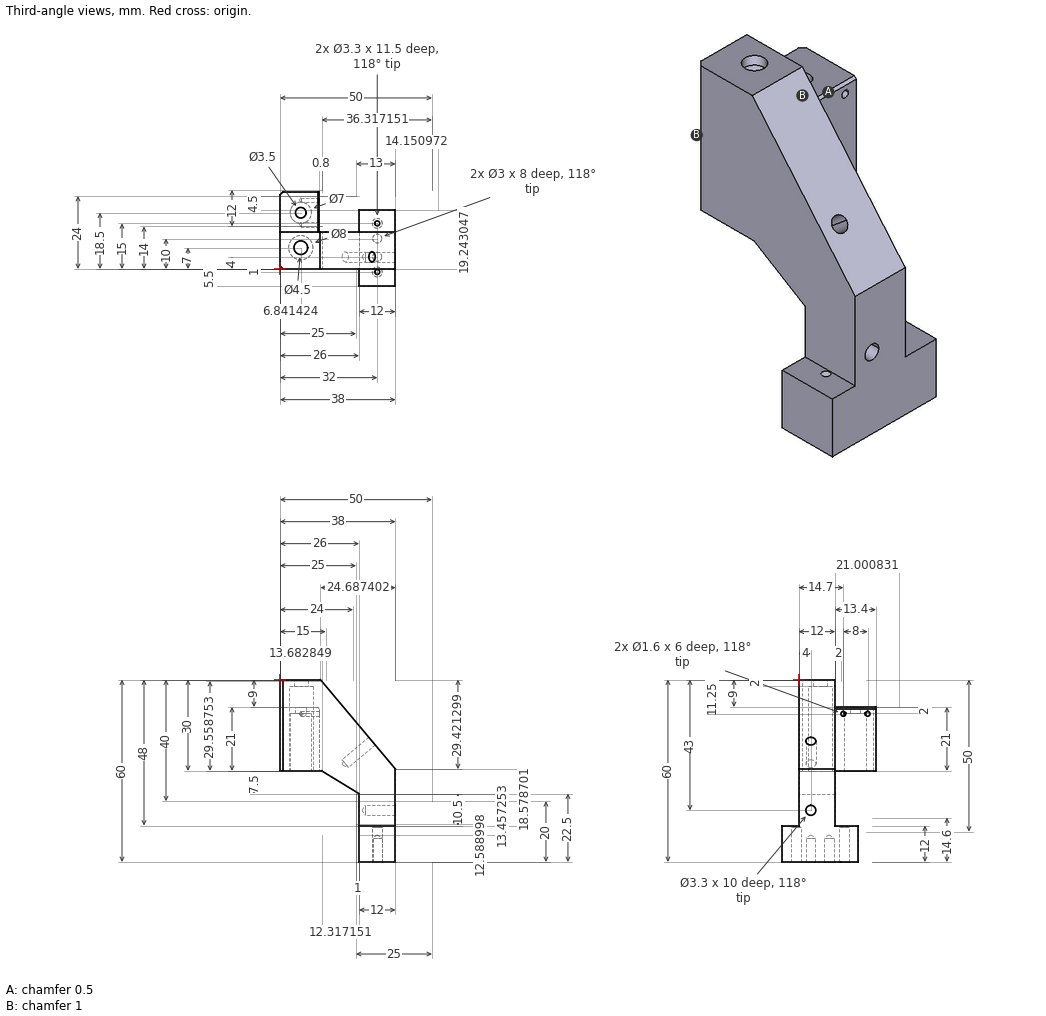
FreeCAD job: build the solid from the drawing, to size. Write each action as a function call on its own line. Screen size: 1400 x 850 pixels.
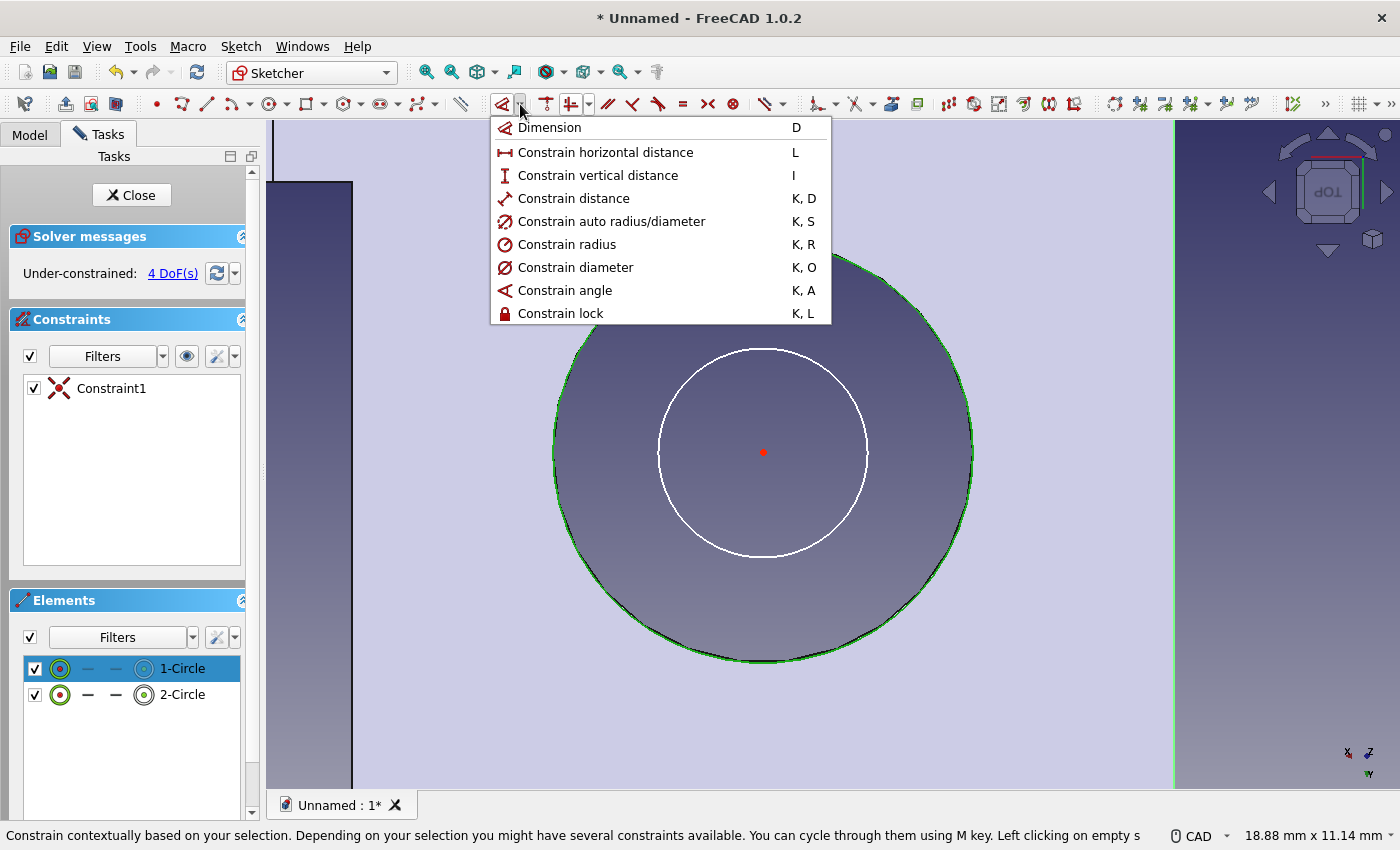
click(661, 268)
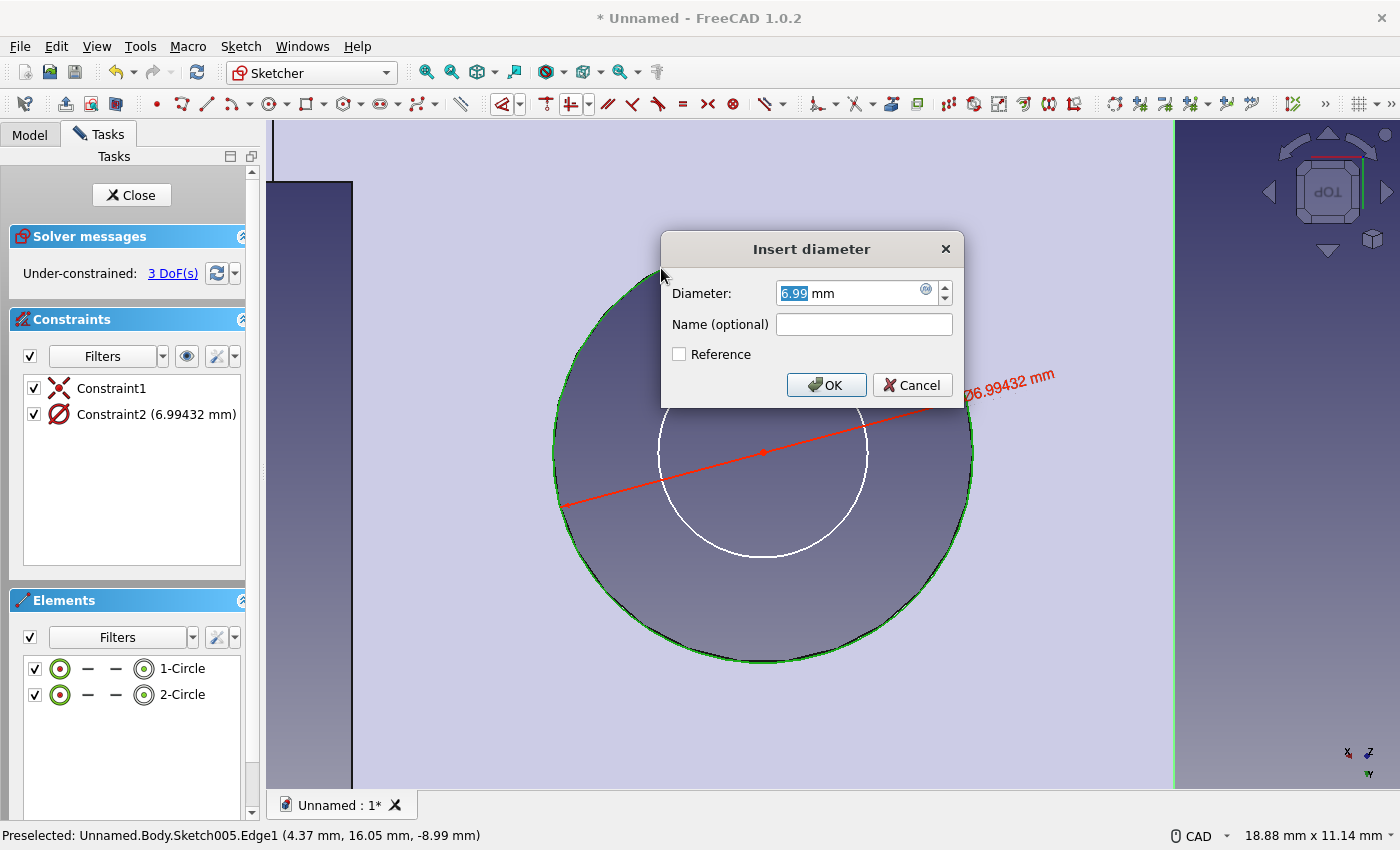
text(7)
key(Return)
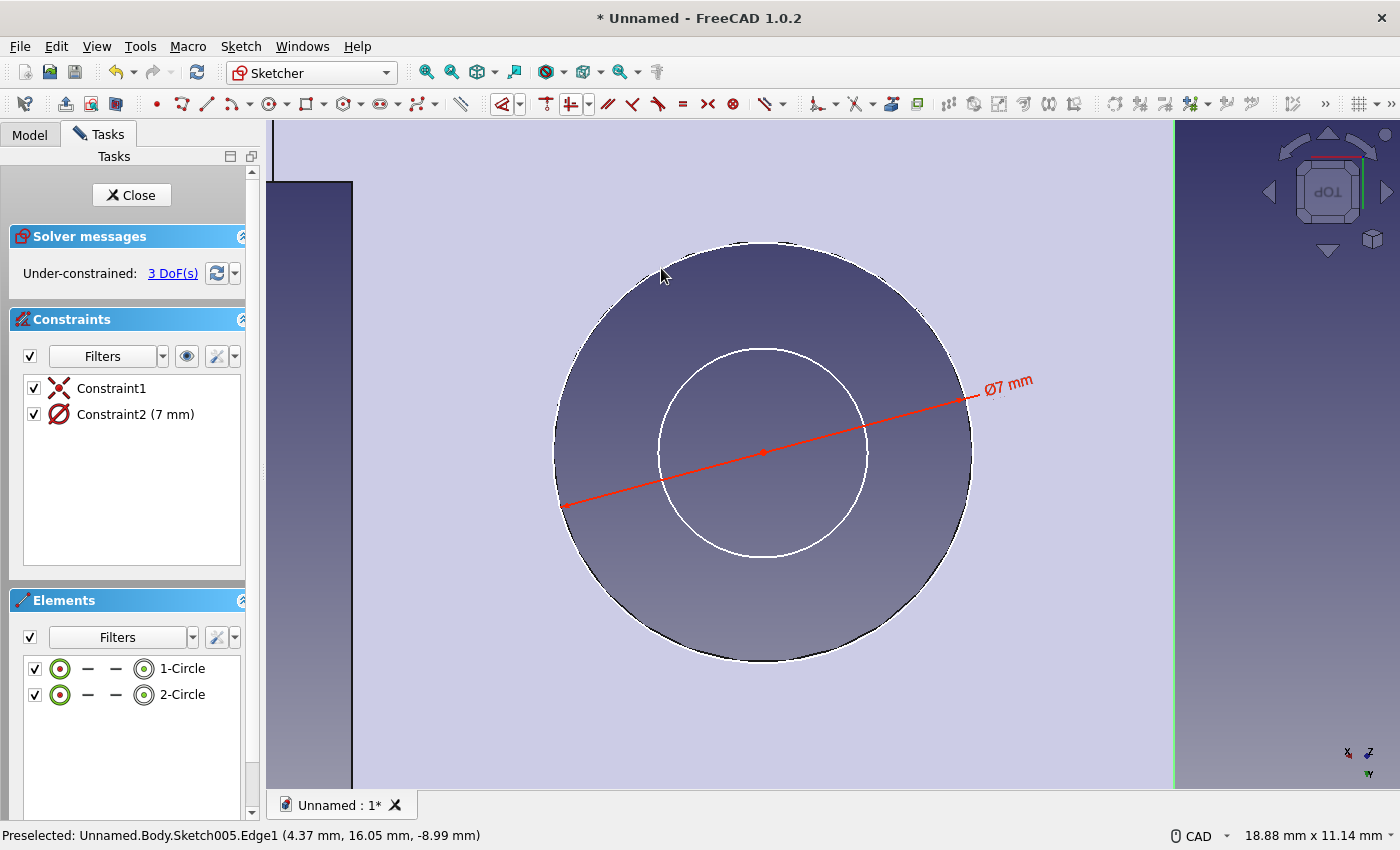
click(837, 379)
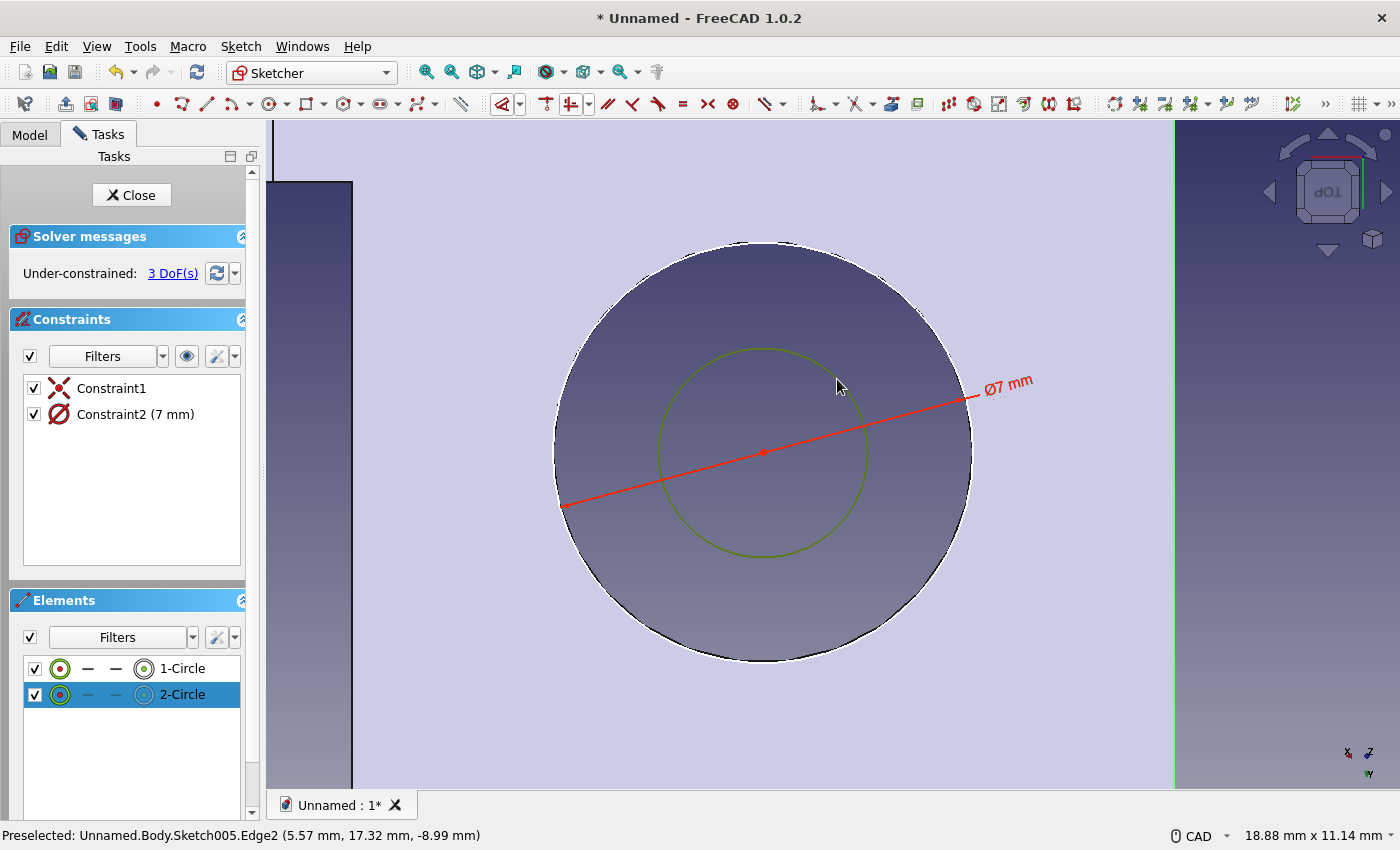
key(k)
key(o)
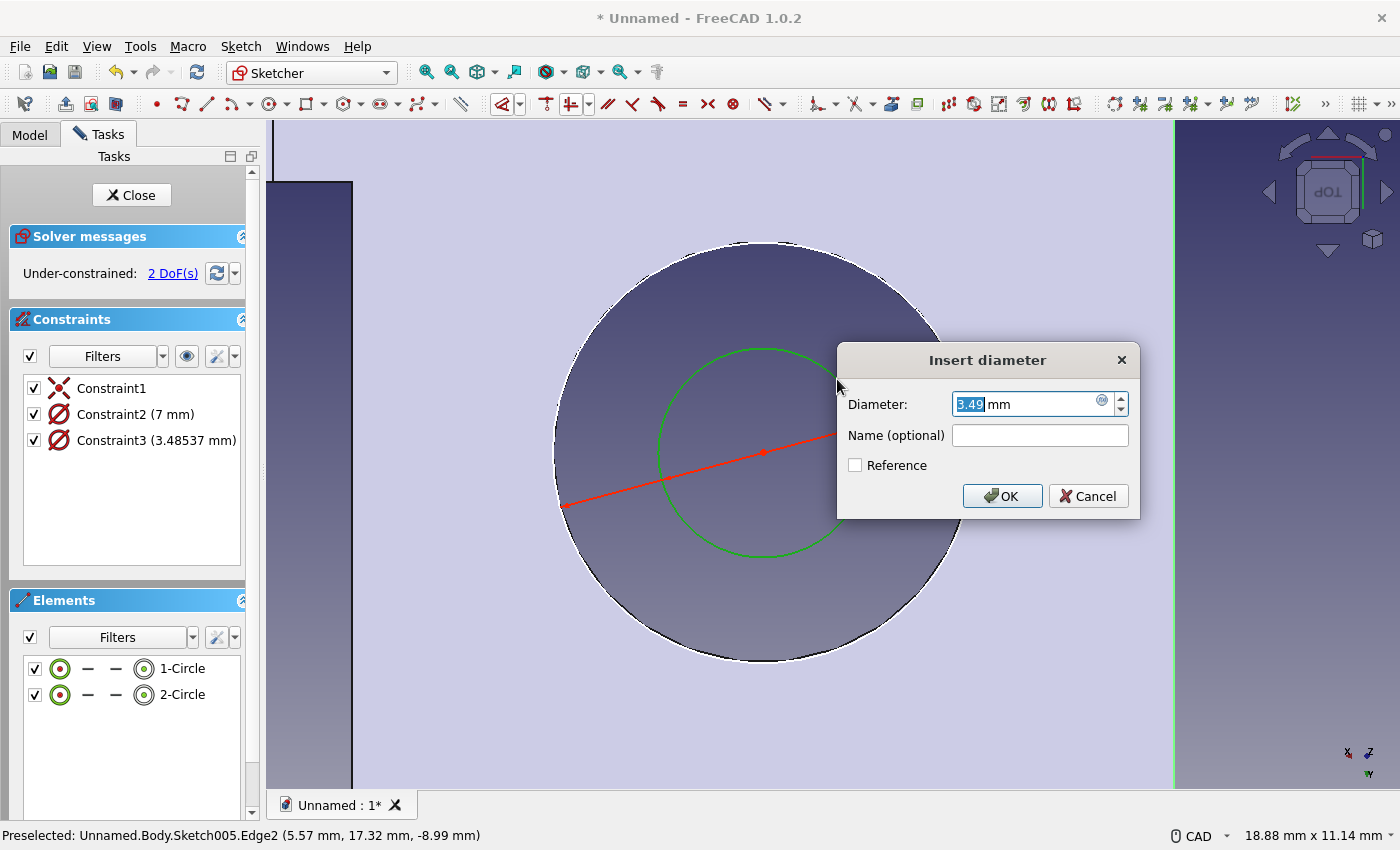
text(3.5)
key(Return)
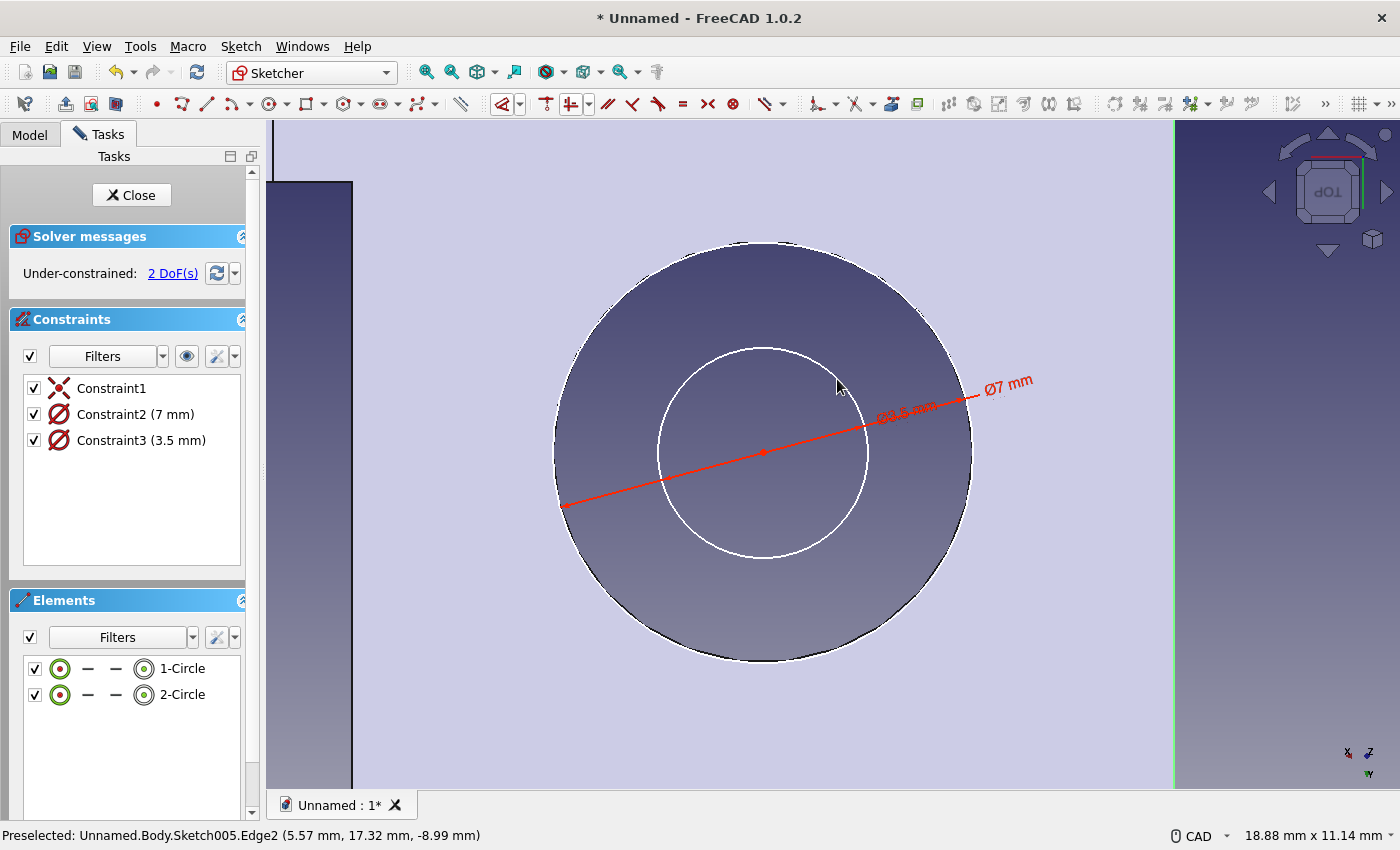
click(763, 453)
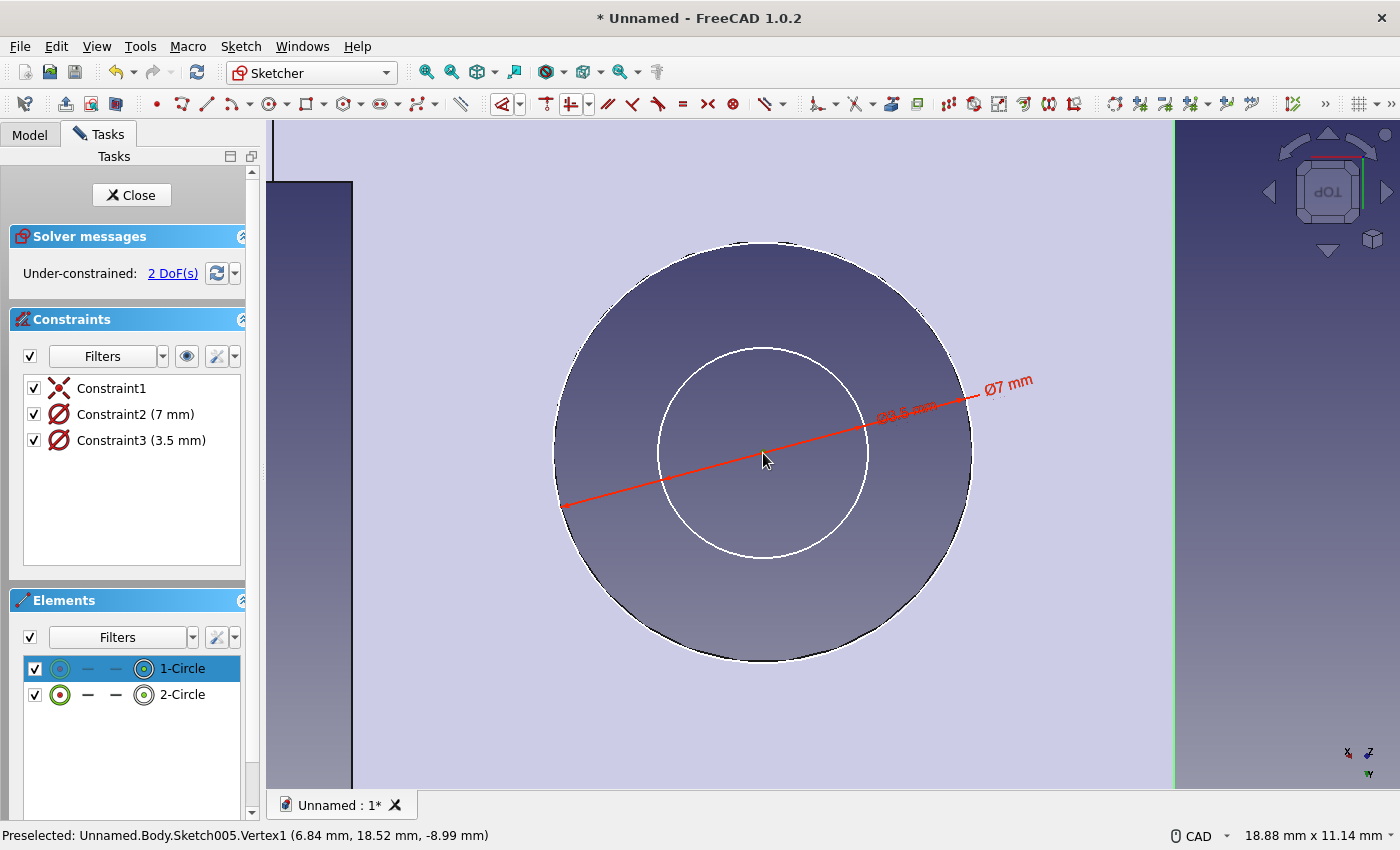
key(i)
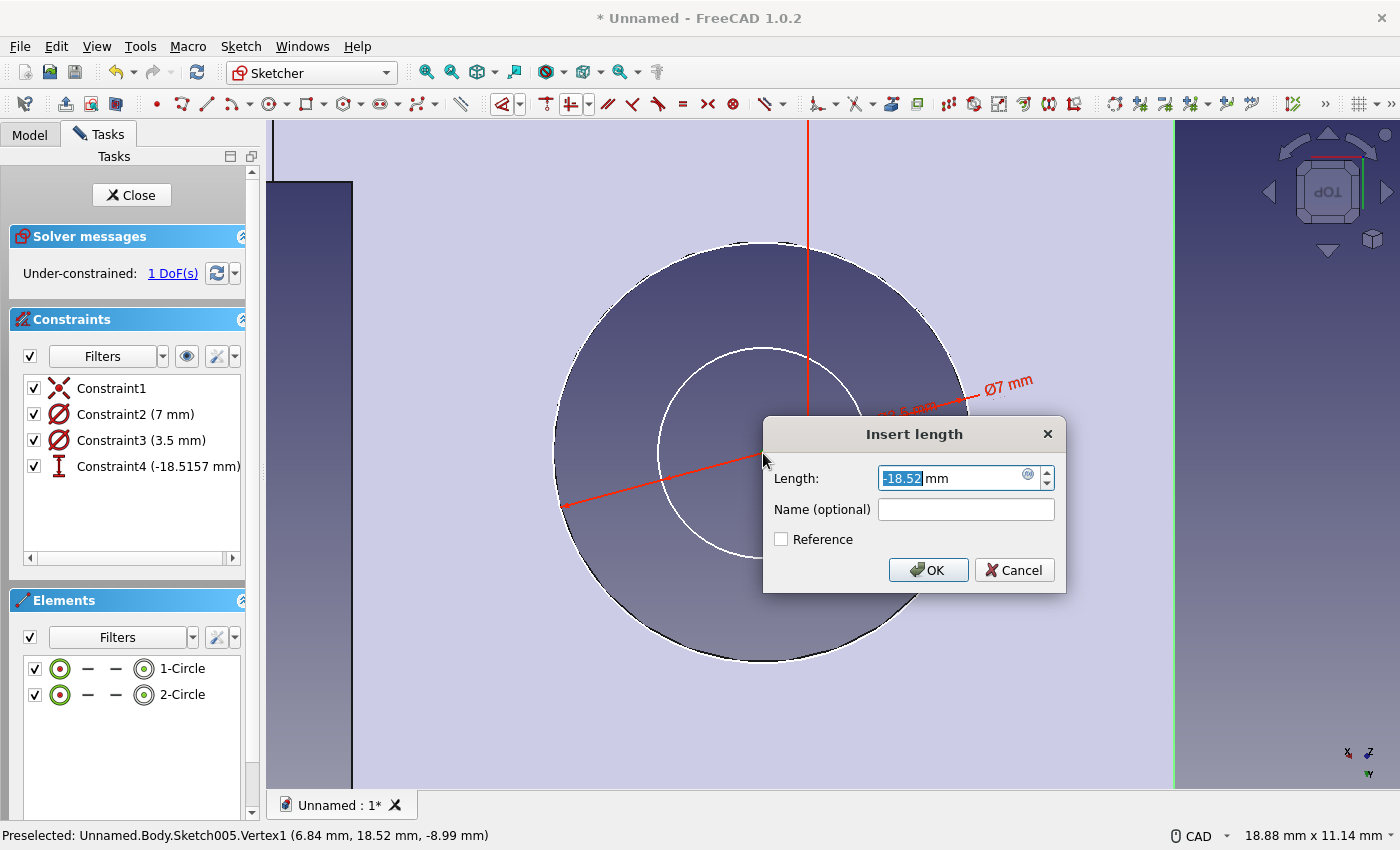
text(-18.5)
key(Return)